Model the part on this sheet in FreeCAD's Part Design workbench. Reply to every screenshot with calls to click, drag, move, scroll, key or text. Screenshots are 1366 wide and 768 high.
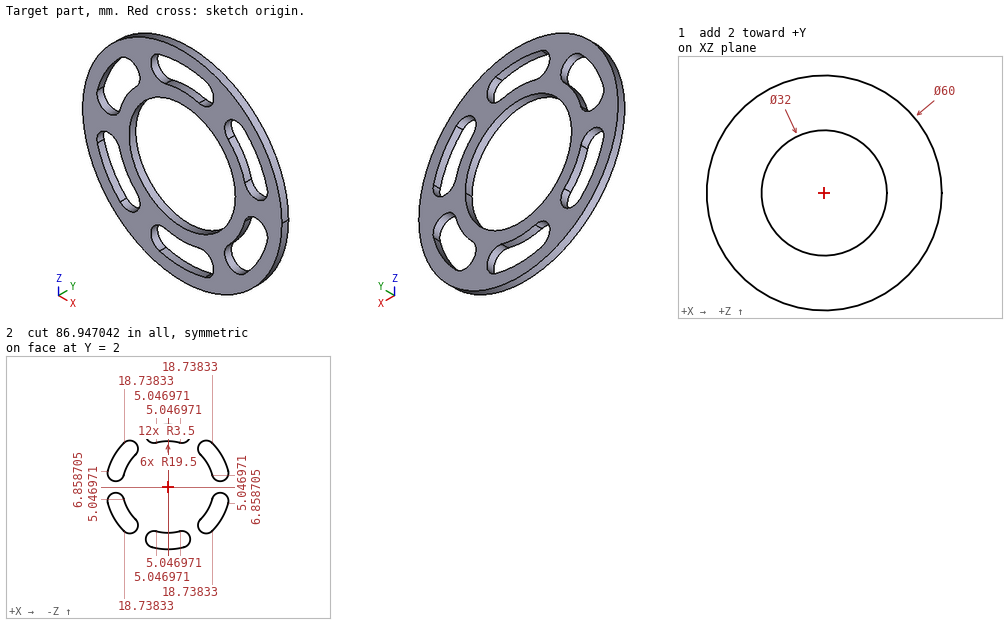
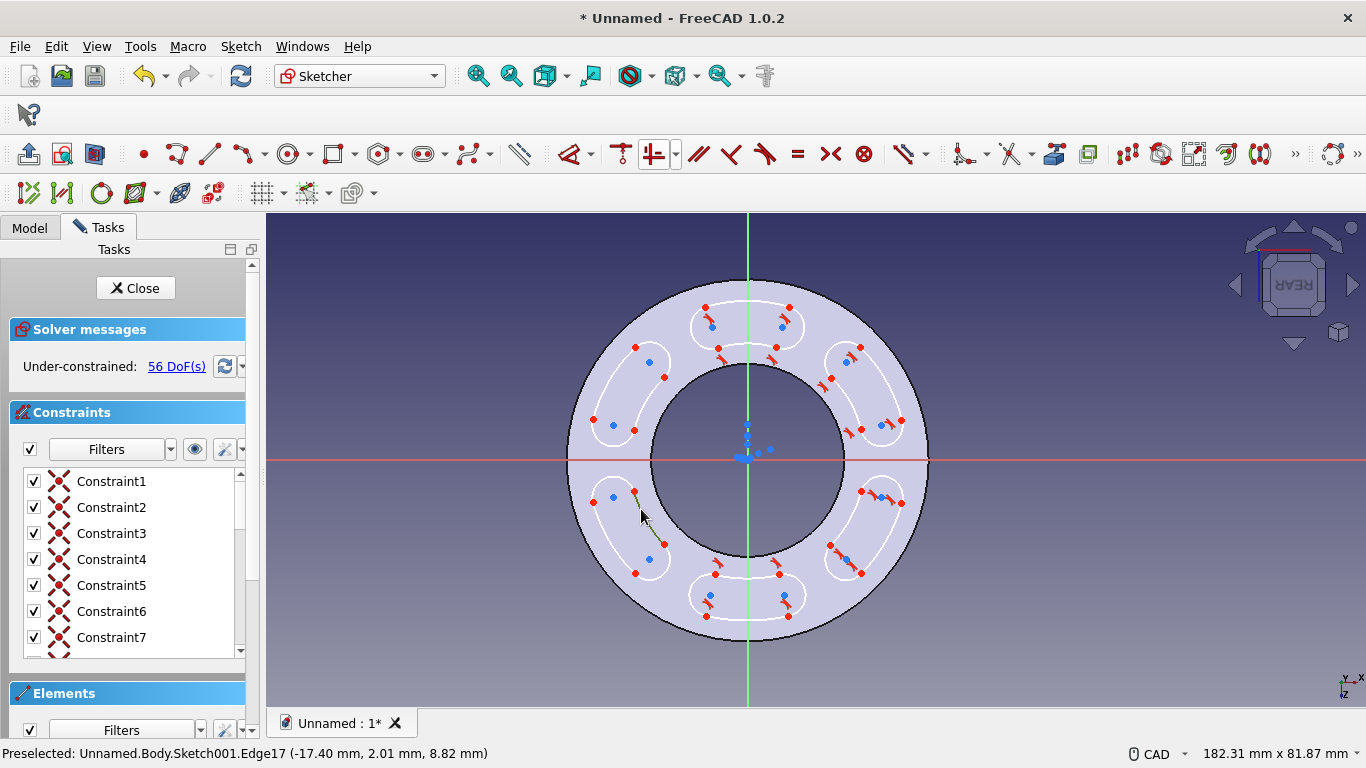
click(621, 478)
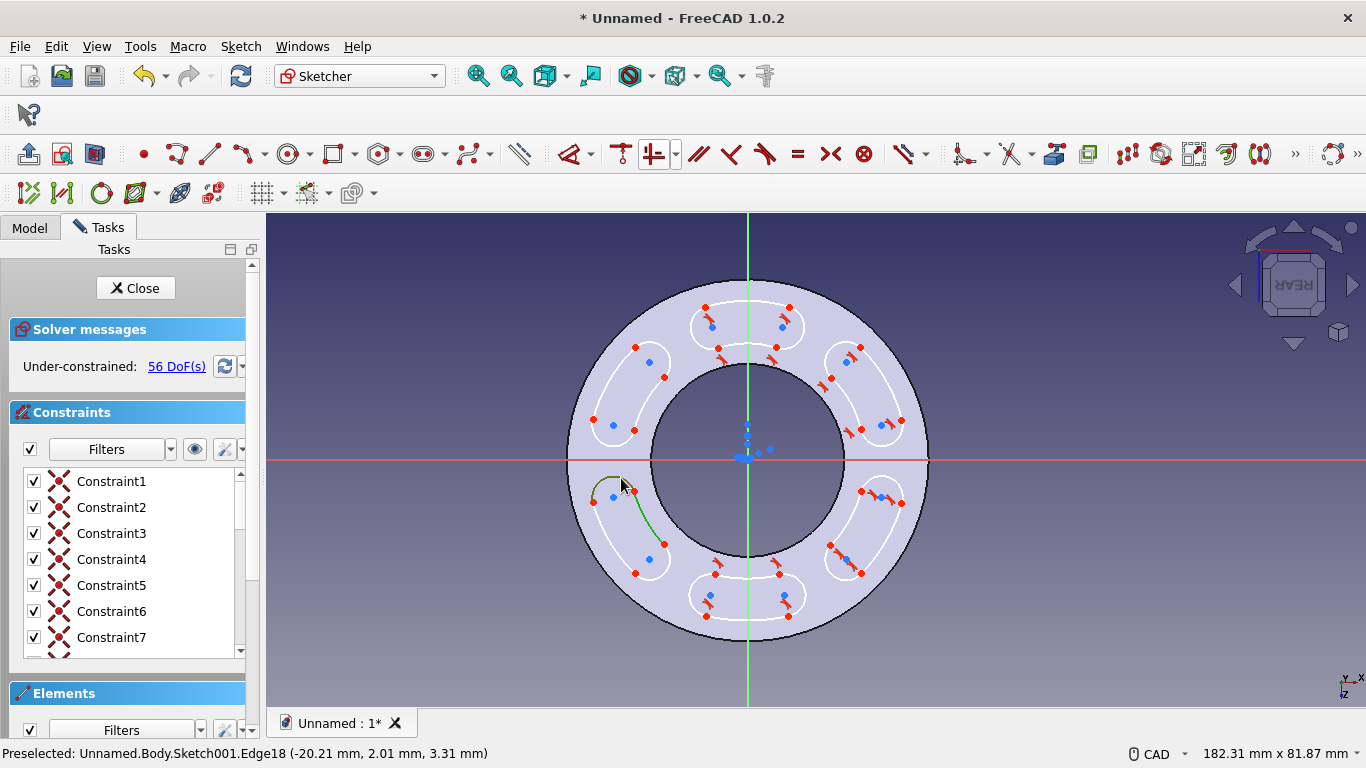
click(765, 154)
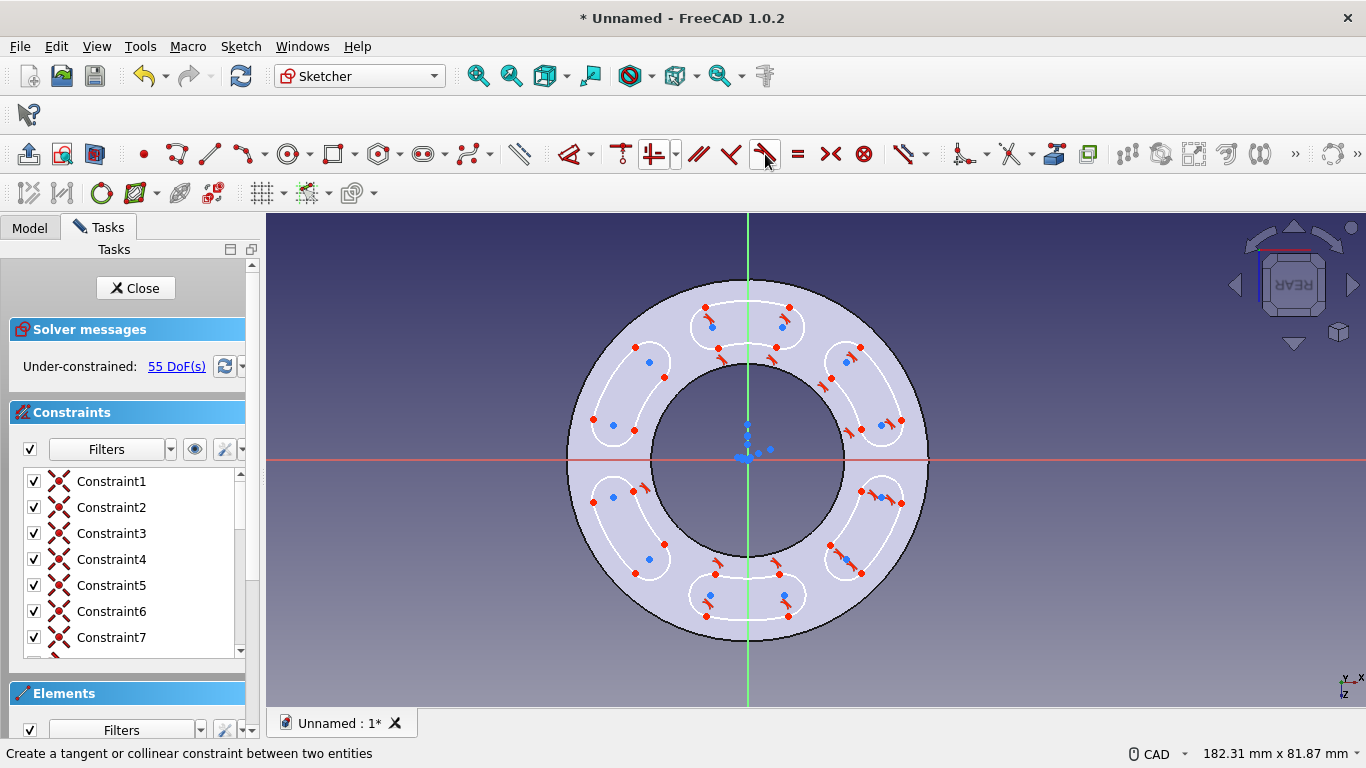
click(640, 509)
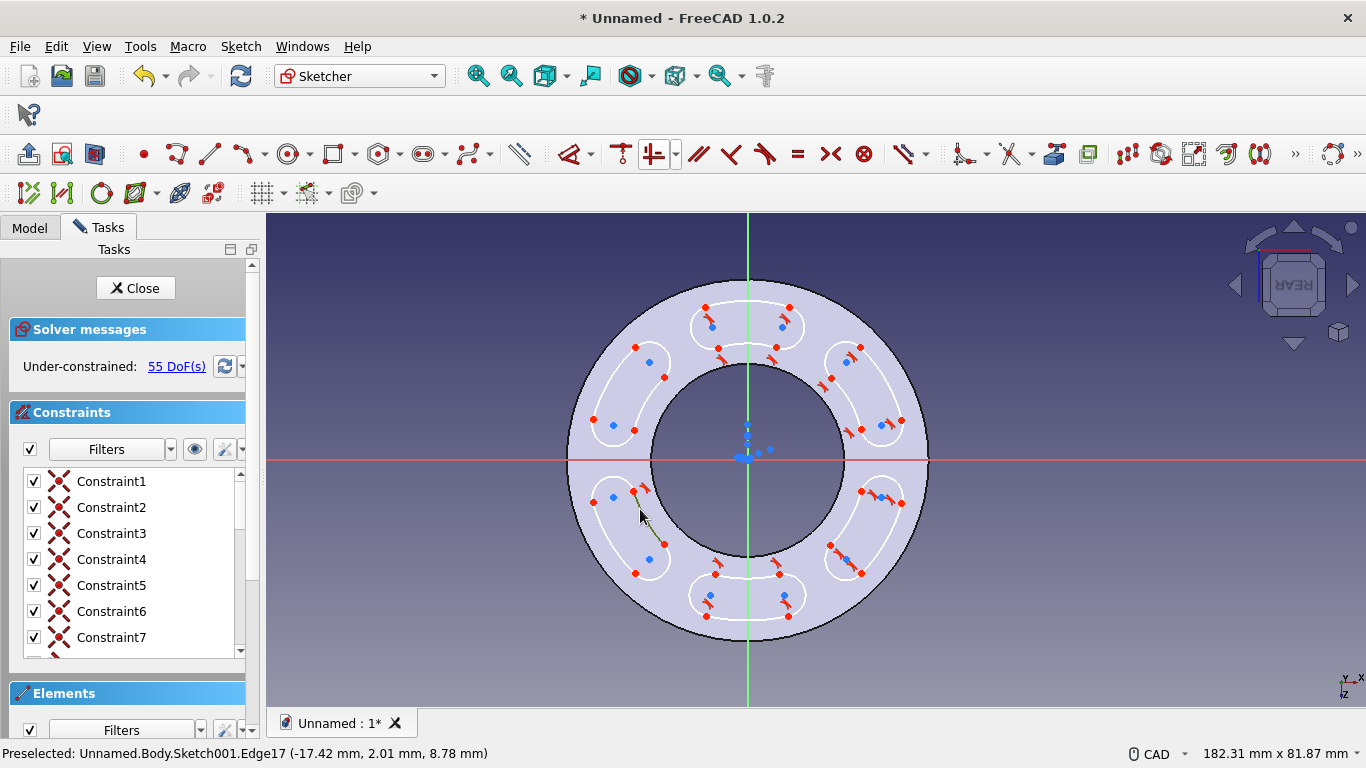
click(653, 580)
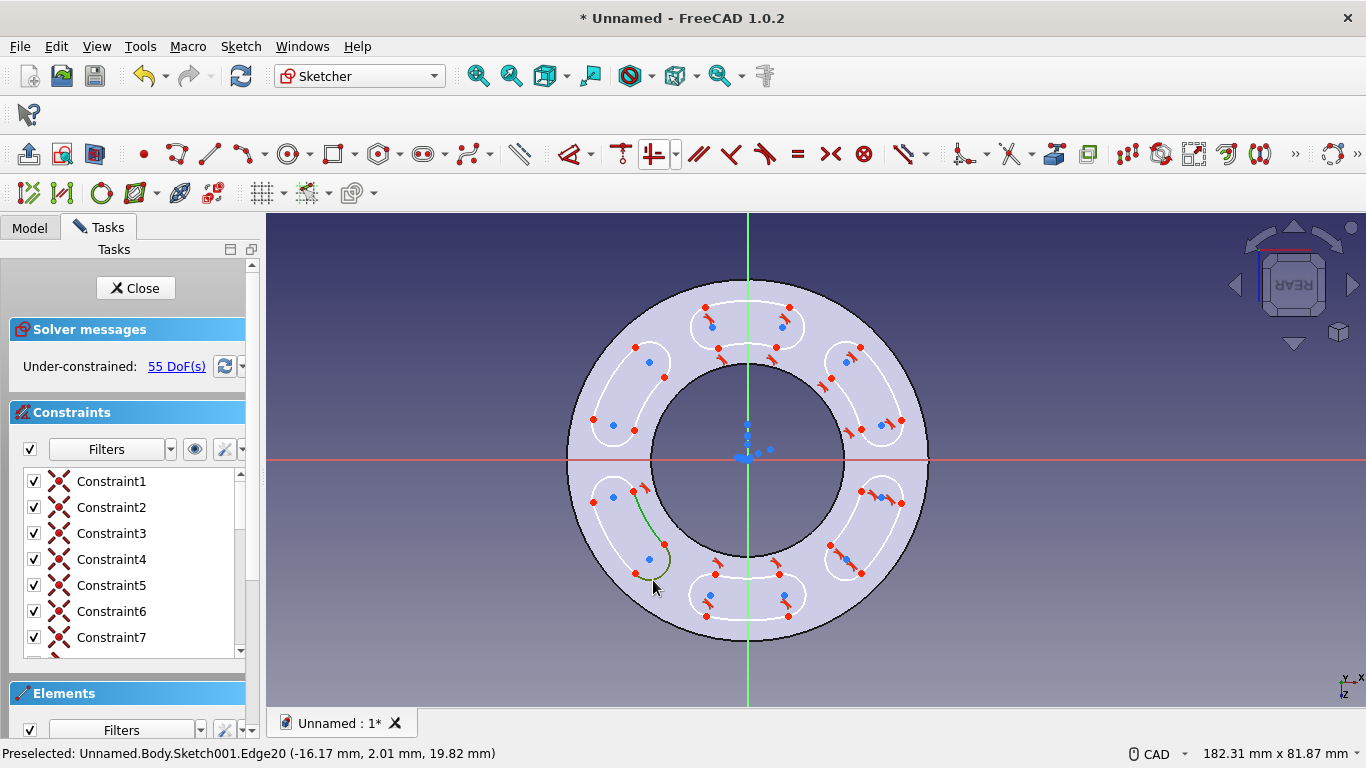
key(t)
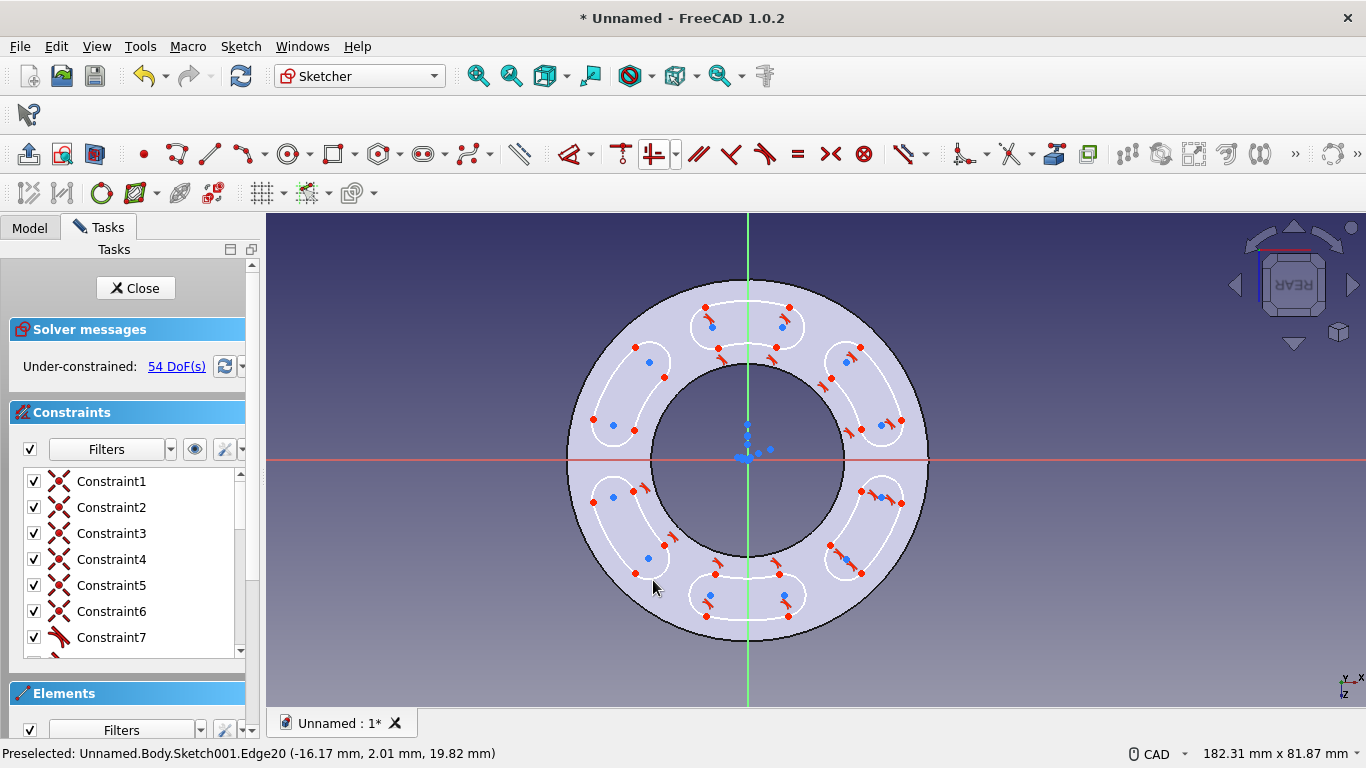
click(621, 478)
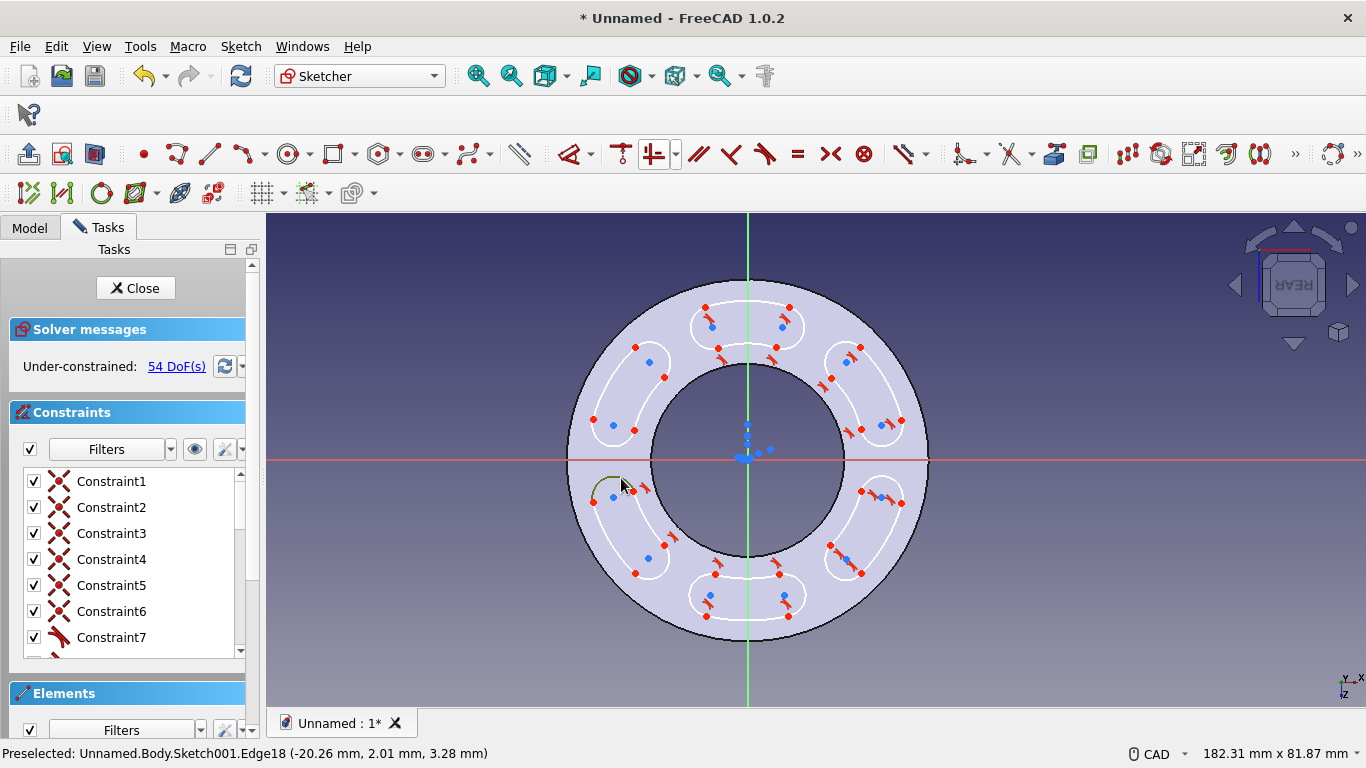
click(602, 526)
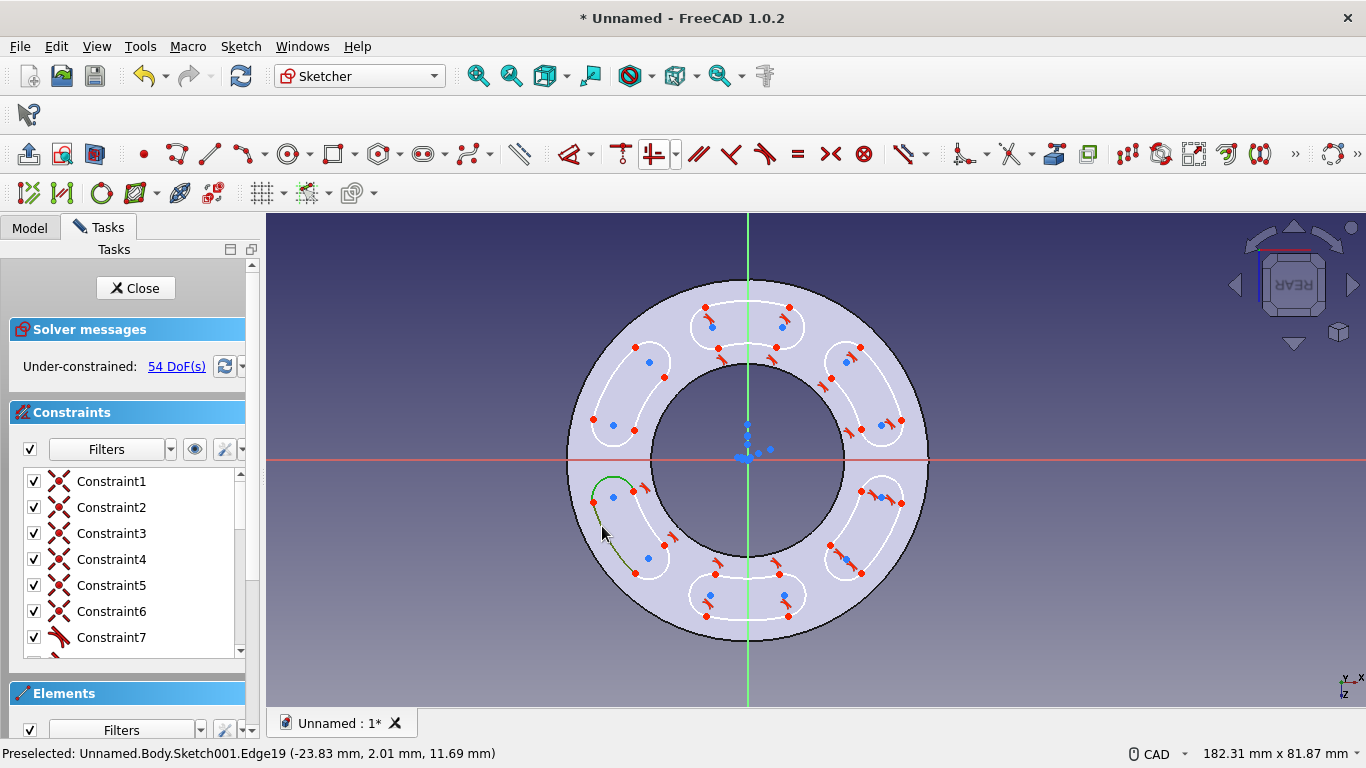
key(t)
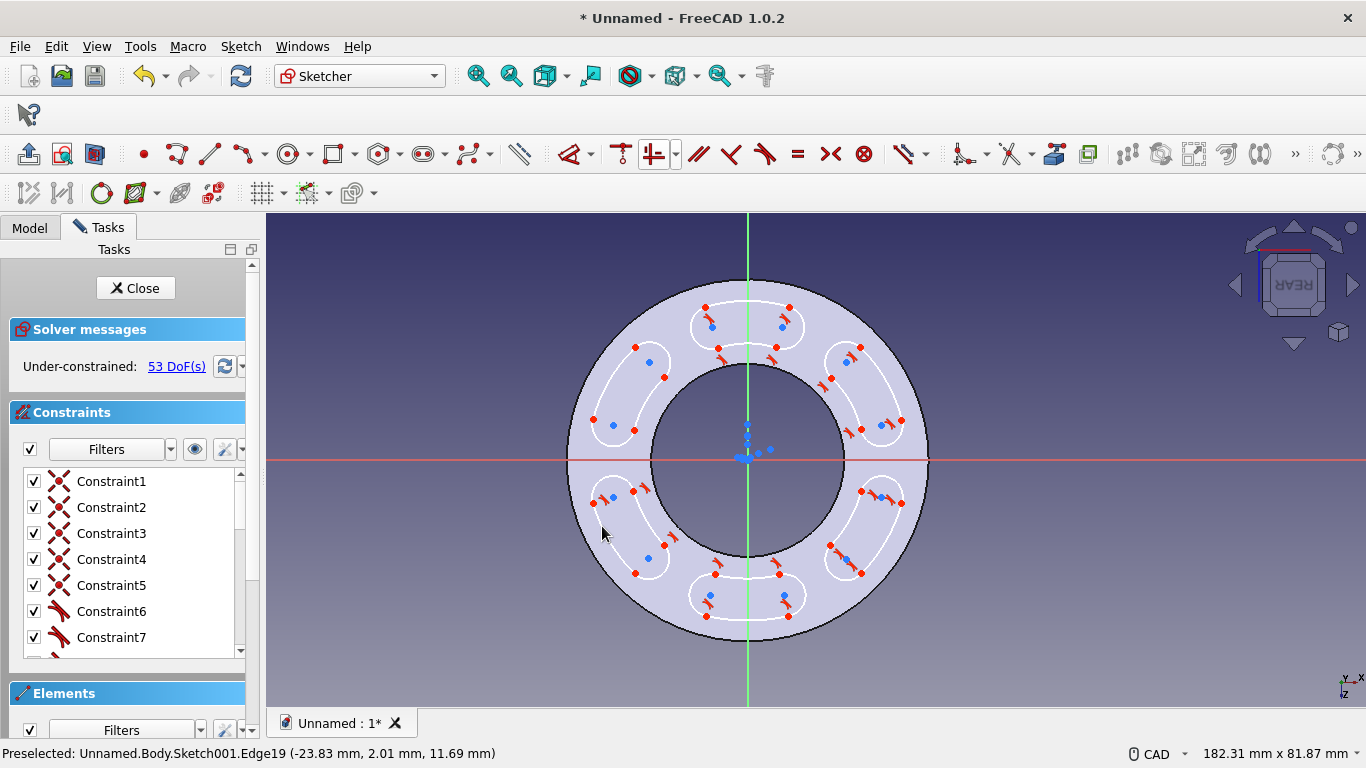
click(602, 526)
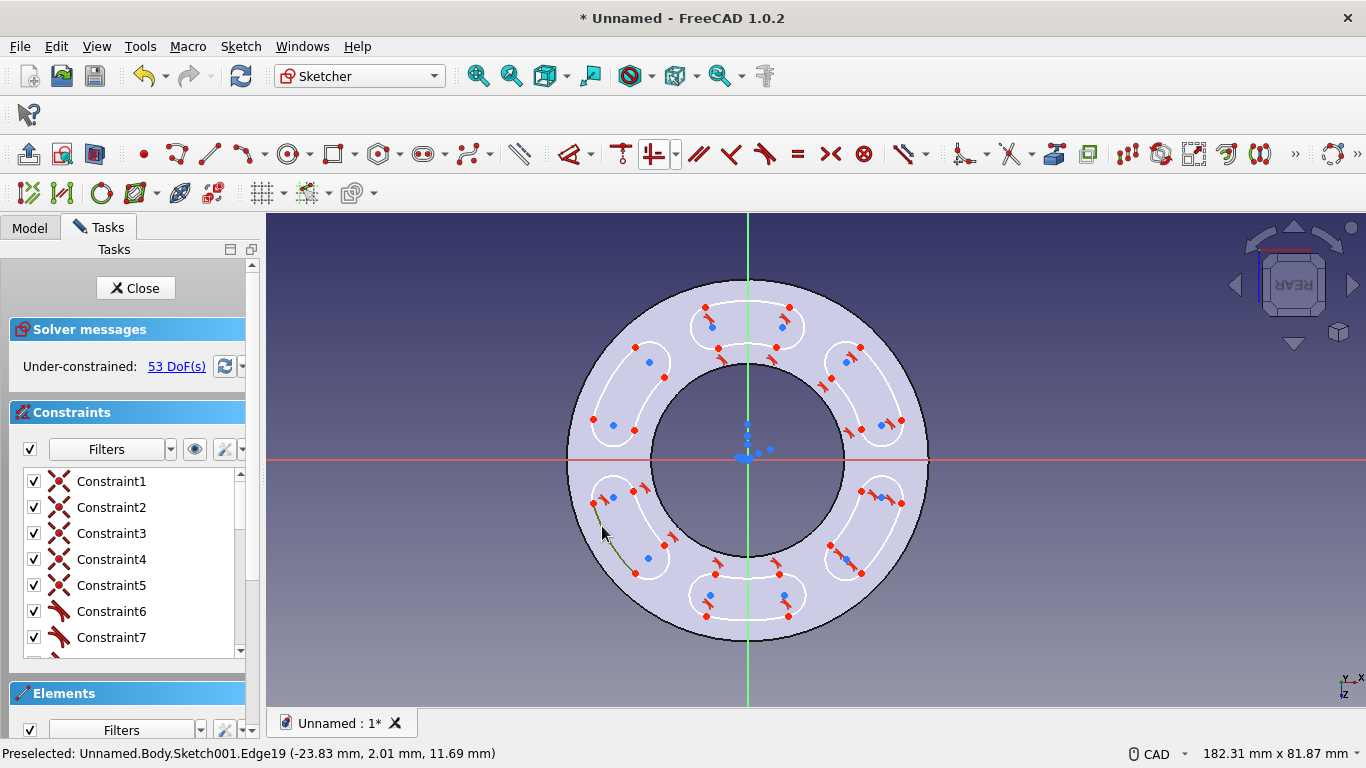
click(652, 579)